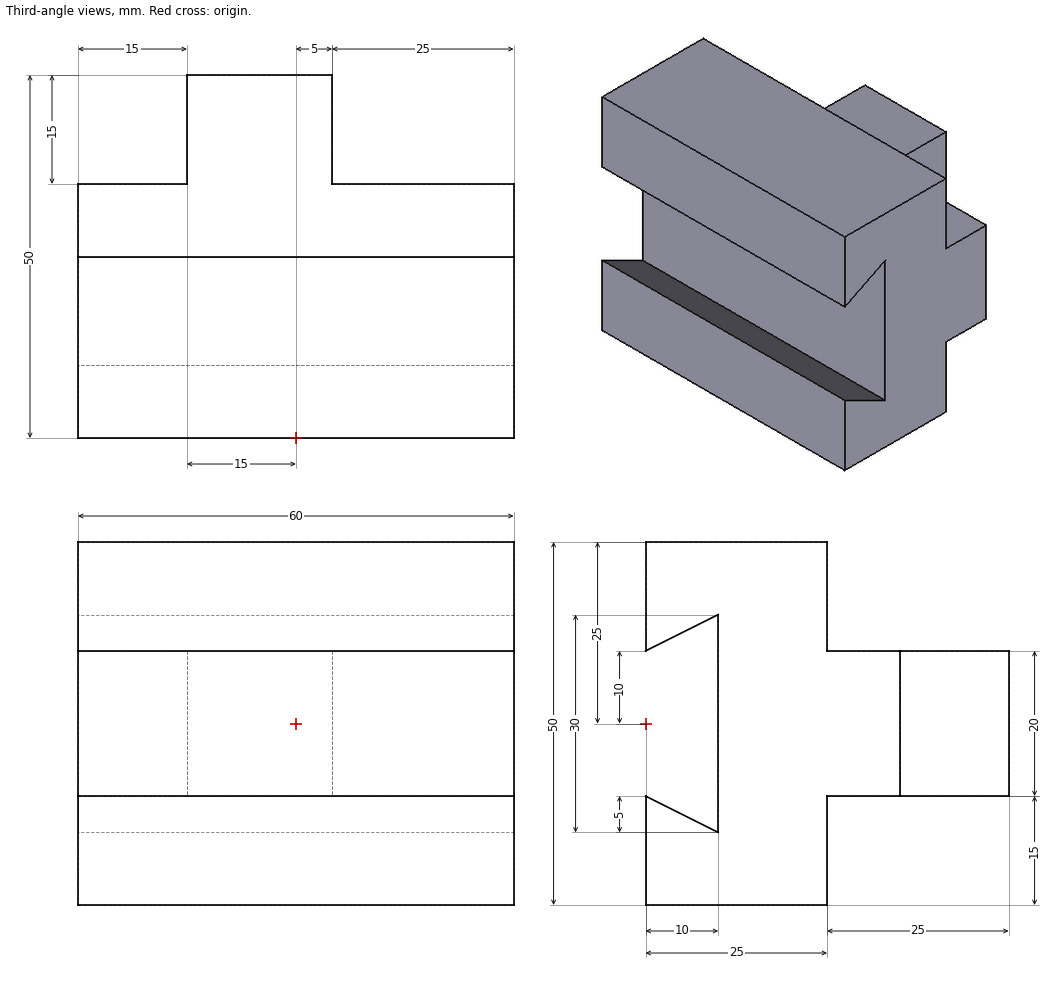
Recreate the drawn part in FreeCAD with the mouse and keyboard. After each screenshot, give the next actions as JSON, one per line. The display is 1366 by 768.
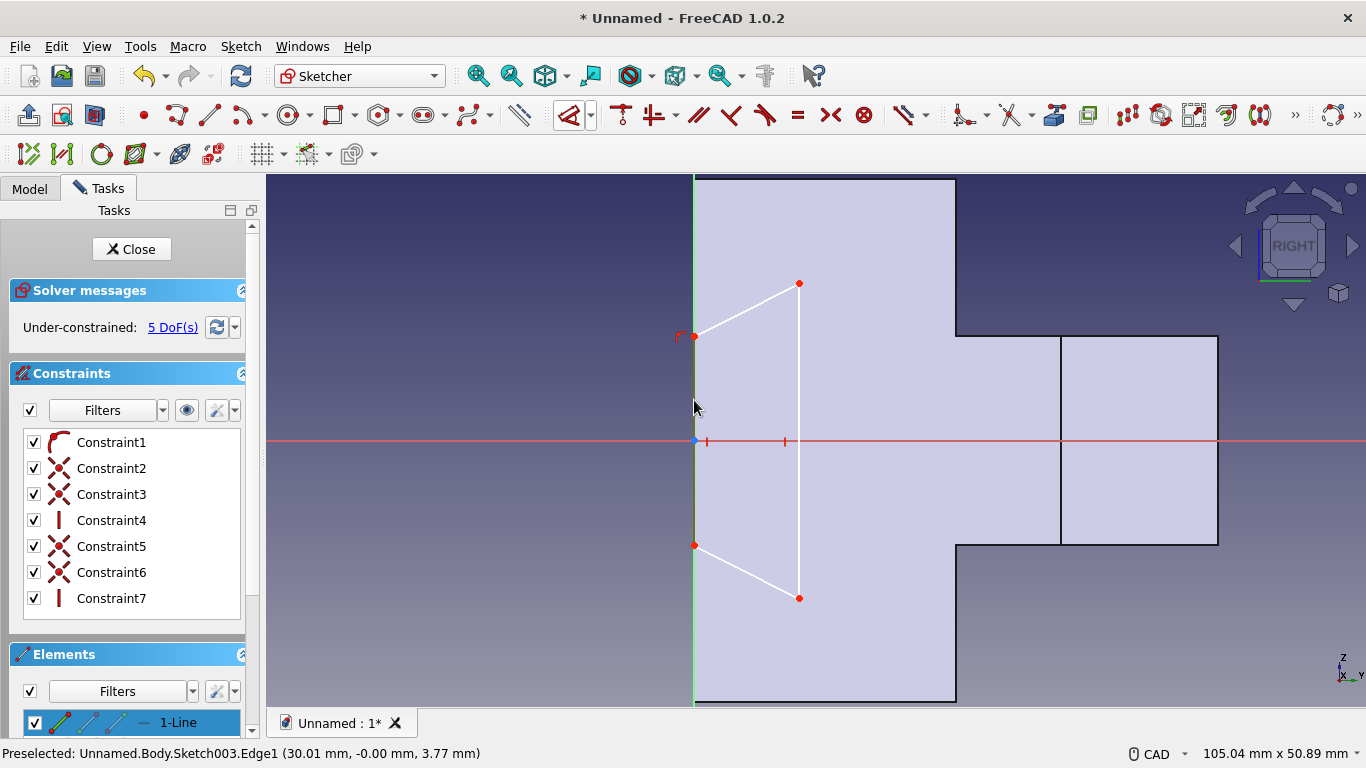
{"action": "key", "text": "i"}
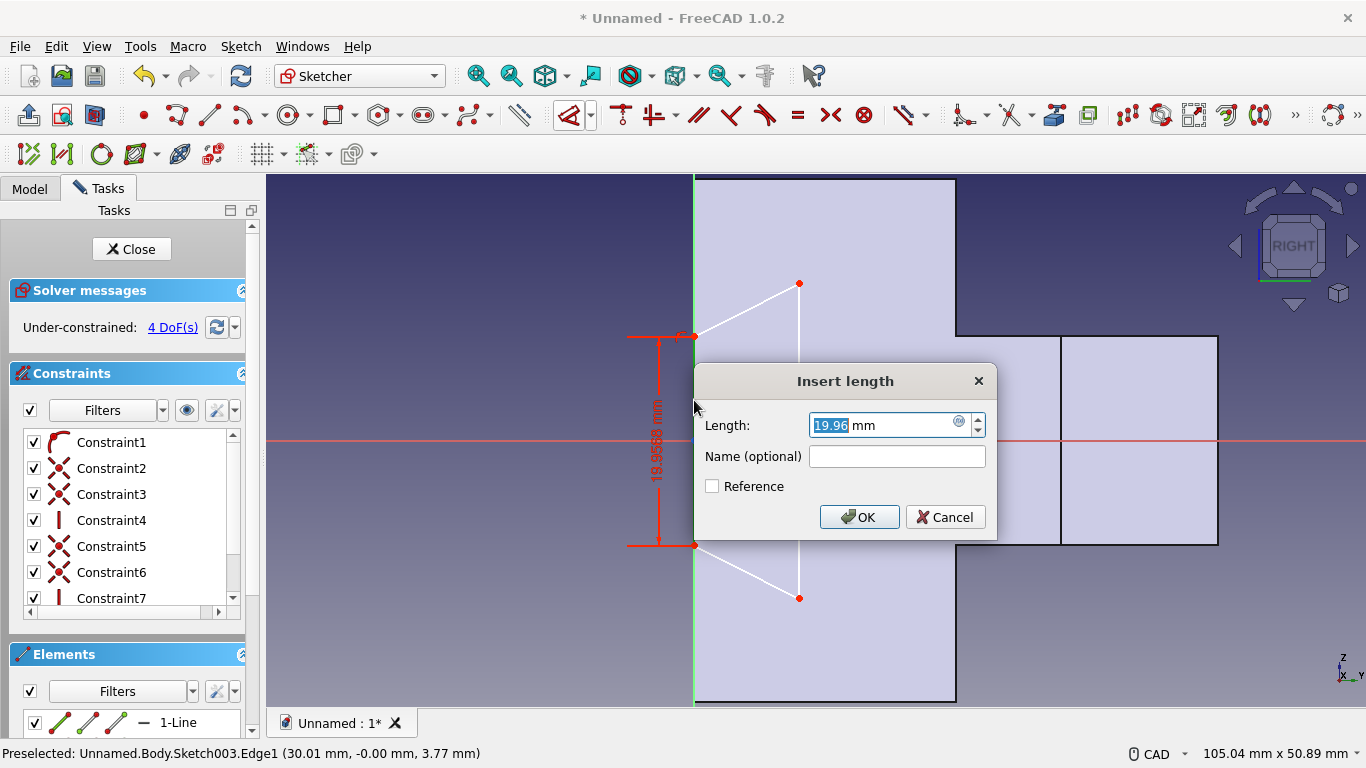
{"action": "type", "text": "20"}
{"action": "key", "text": "Return"}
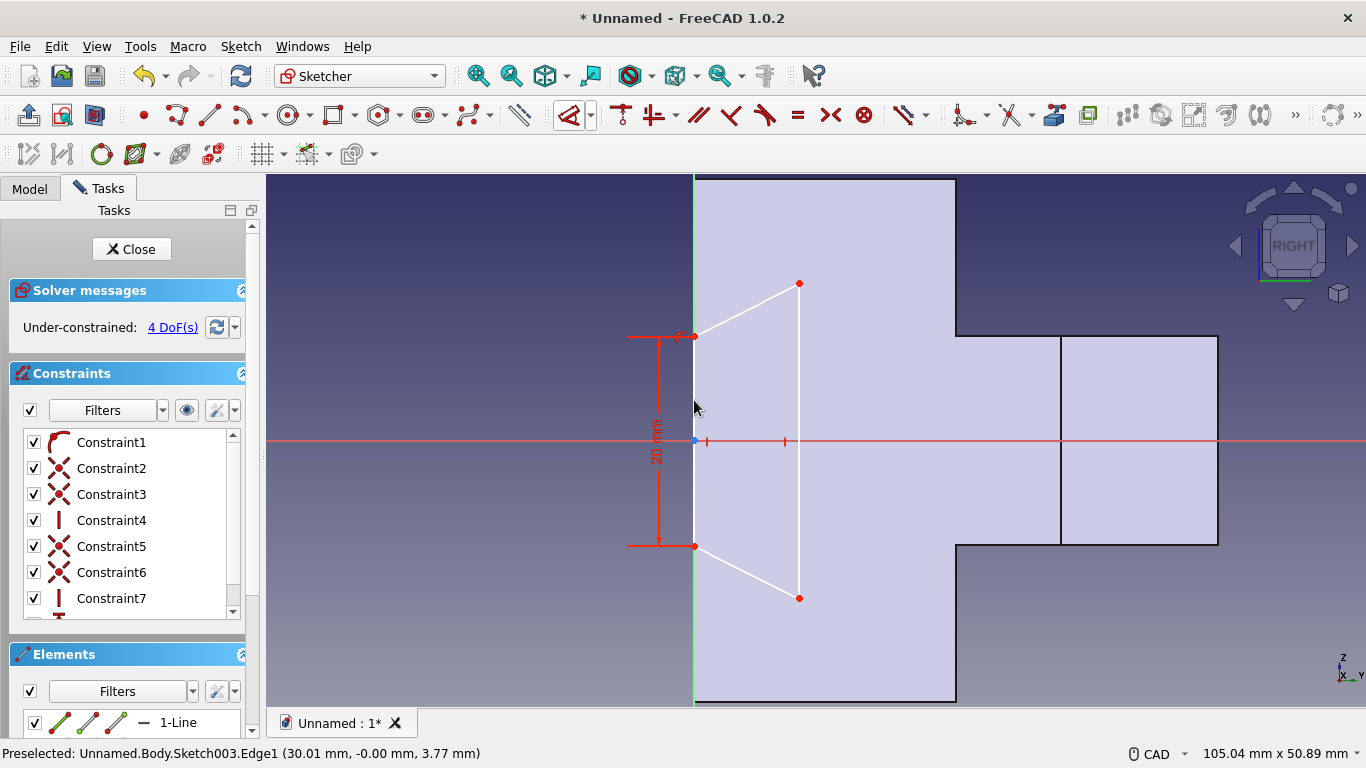
{"action": "left_click", "coordinate": [799, 505]}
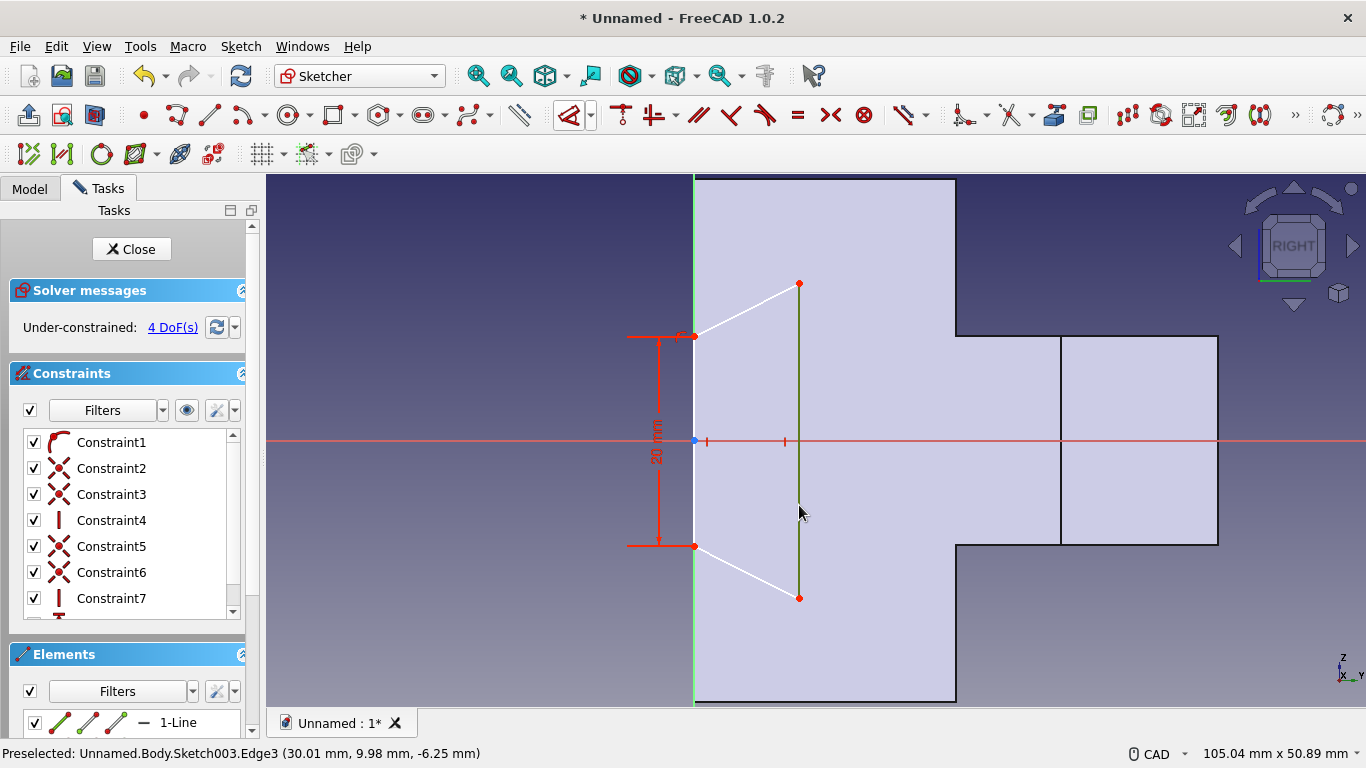
{"action": "key", "text": "i"}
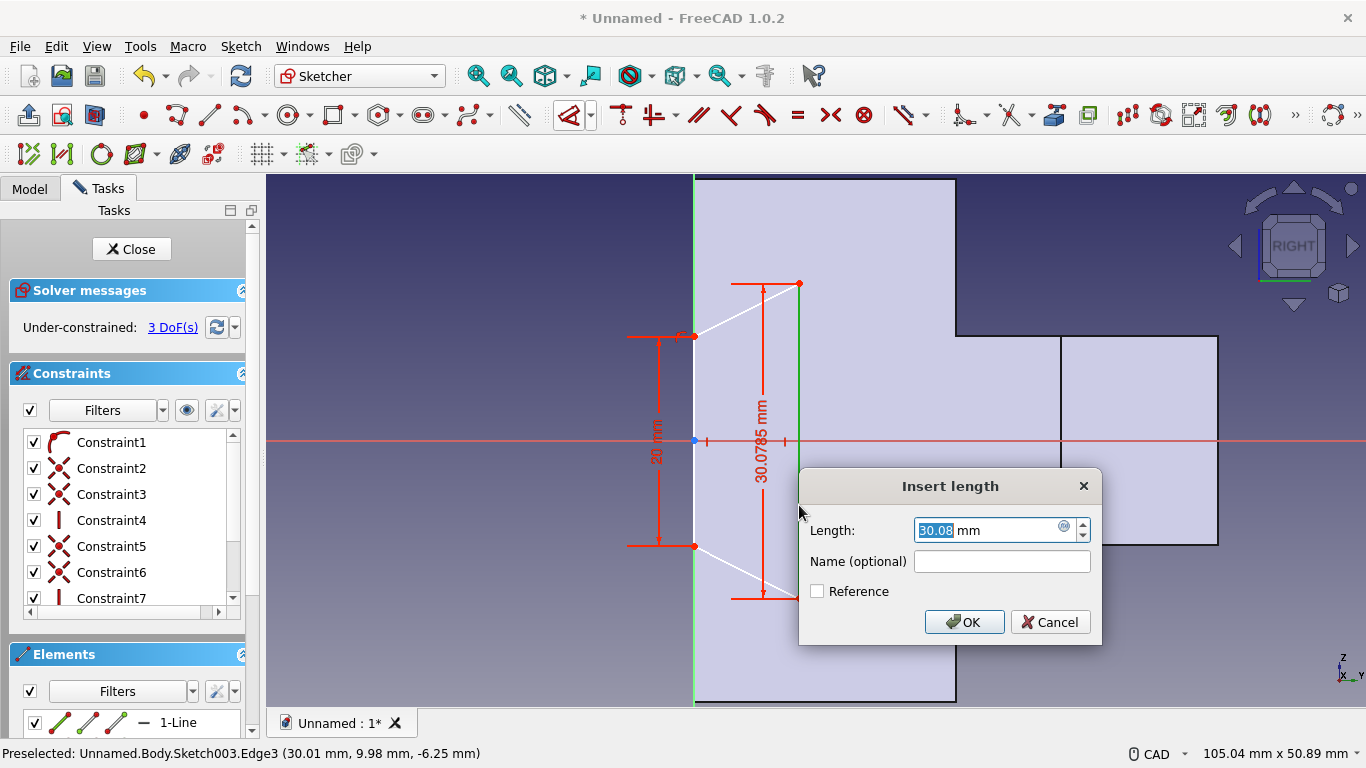
{"action": "type", "text": "30"}
{"action": "key", "text": "Return"}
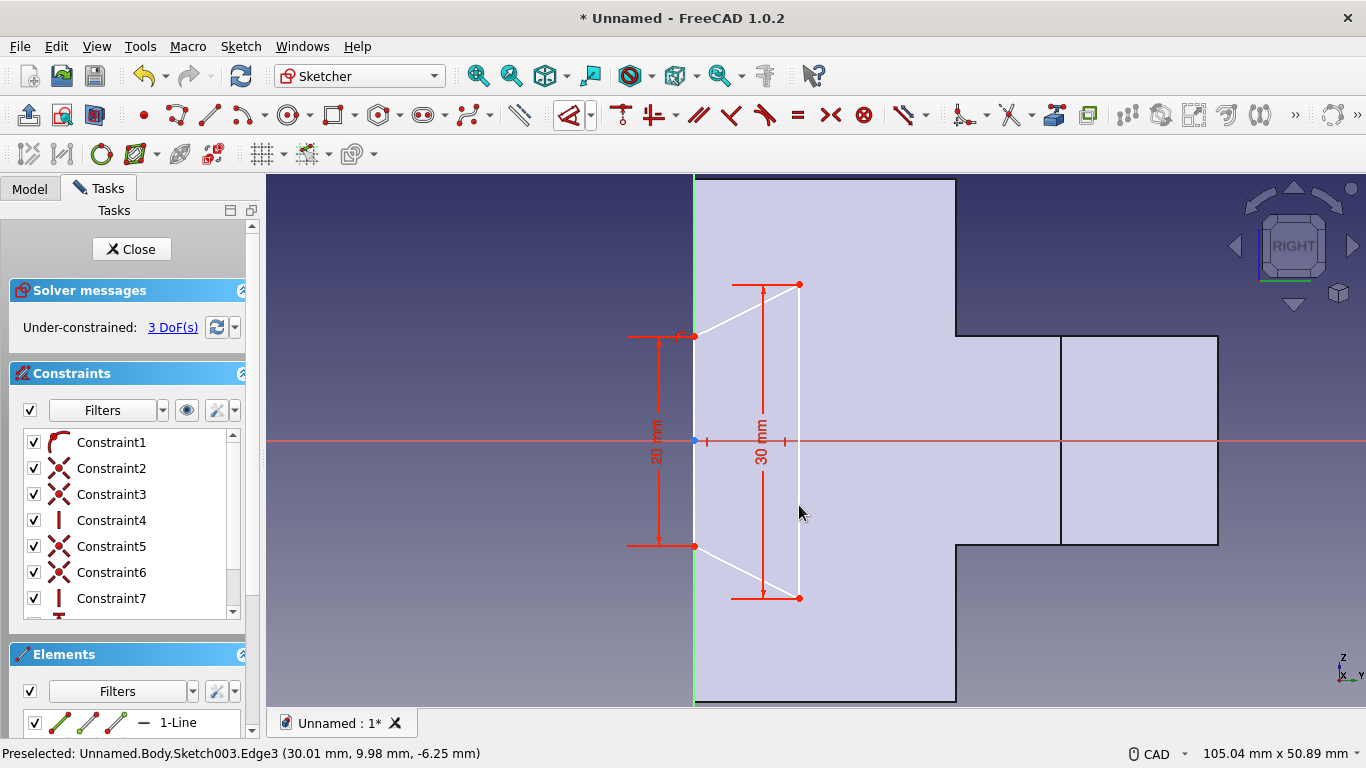
{"action": "left_click", "coordinate": [726, 562]}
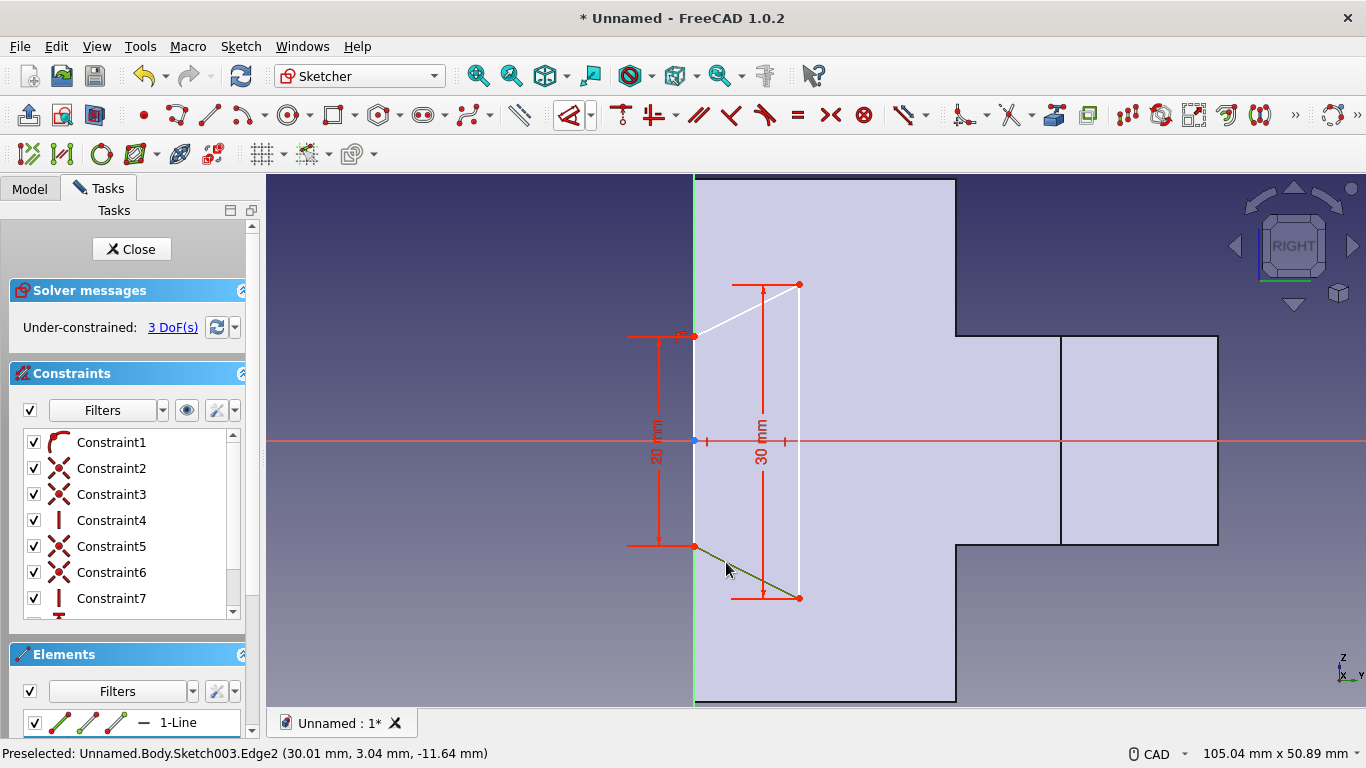
{"action": "left_click", "coordinate": [590, 116]}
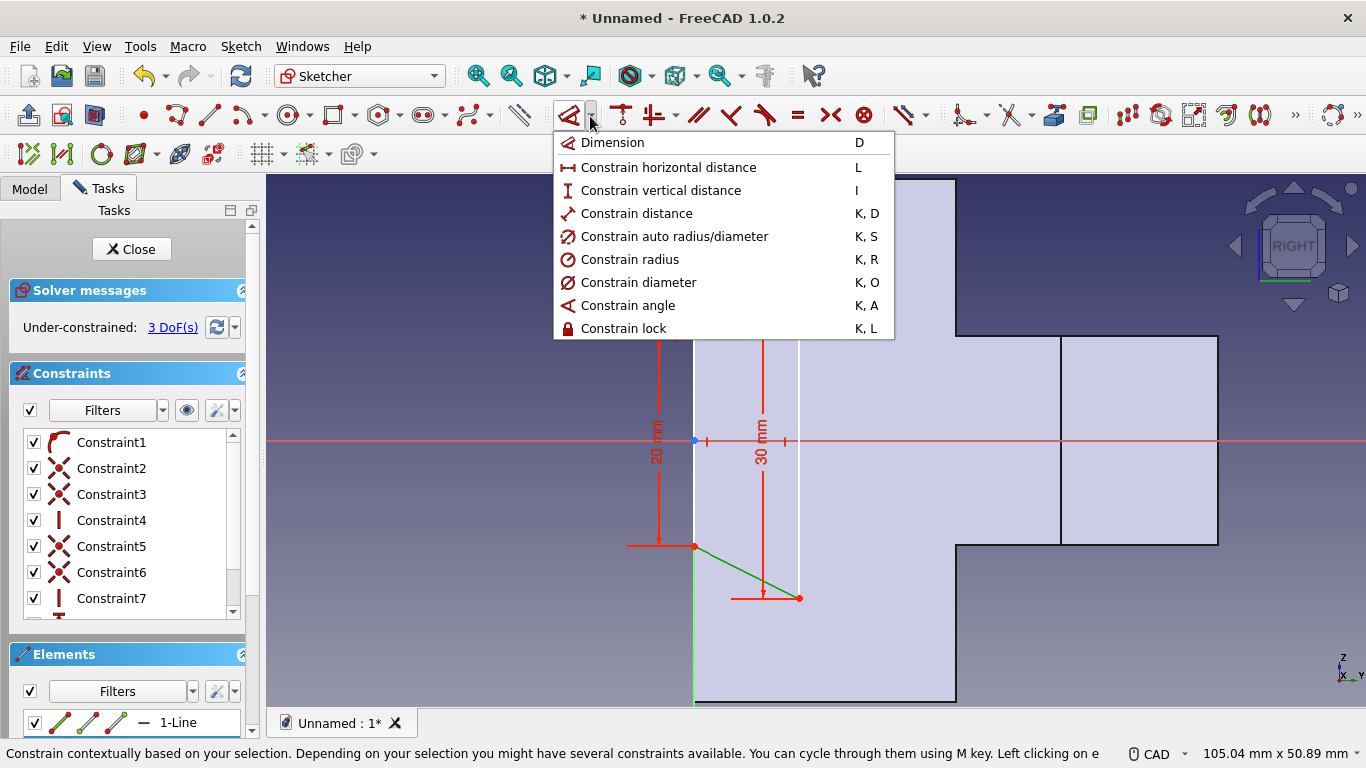
{"action": "left_click", "coordinate": [724, 190]}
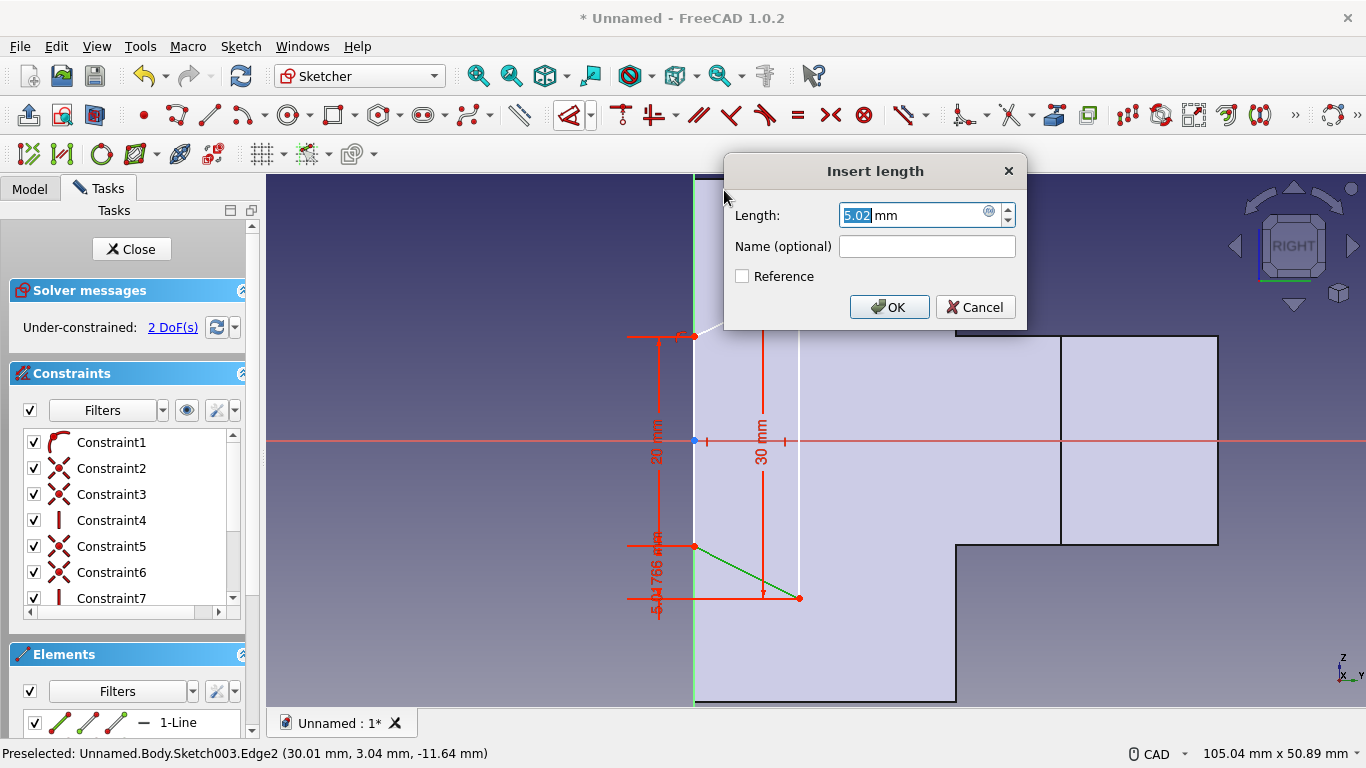
{"action": "type", "text": "5"}
{"action": "key", "text": "Return"}